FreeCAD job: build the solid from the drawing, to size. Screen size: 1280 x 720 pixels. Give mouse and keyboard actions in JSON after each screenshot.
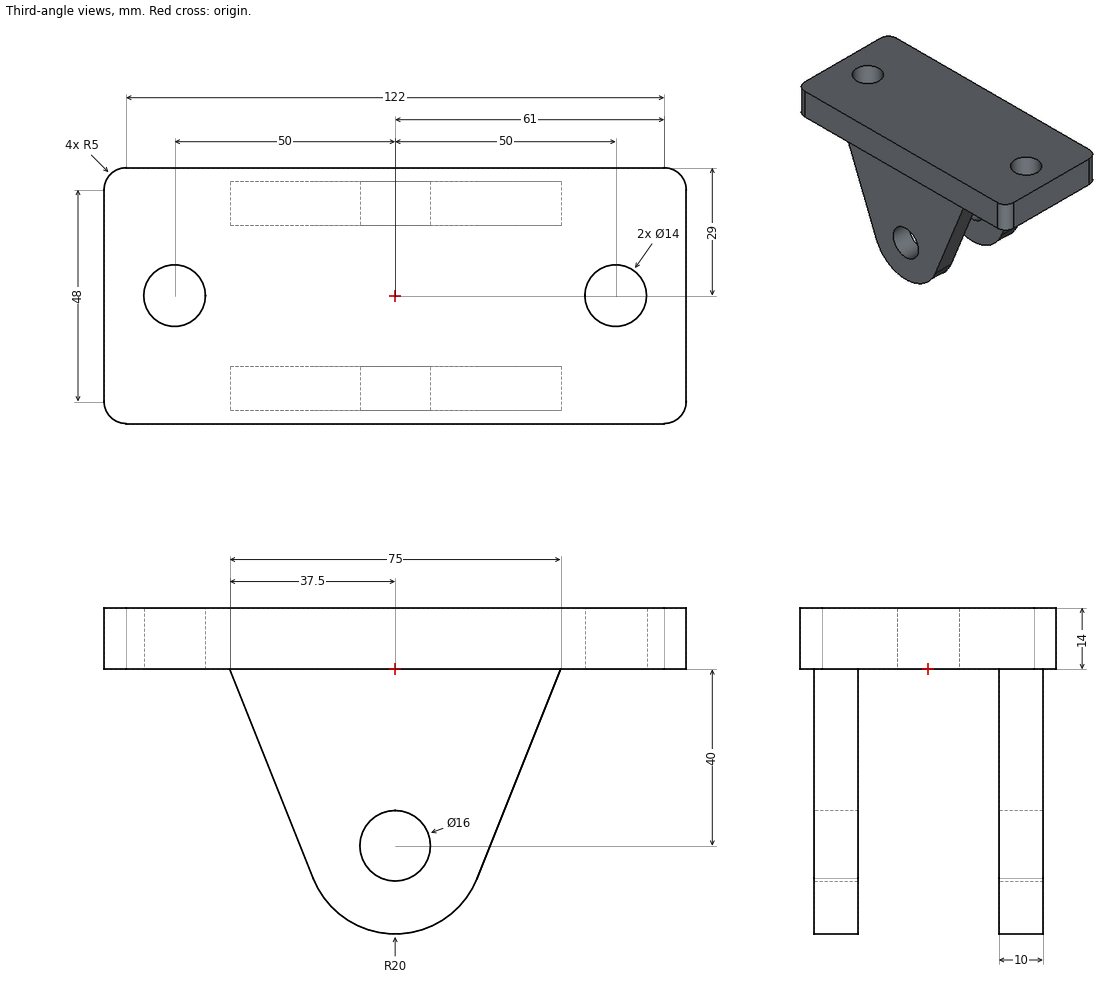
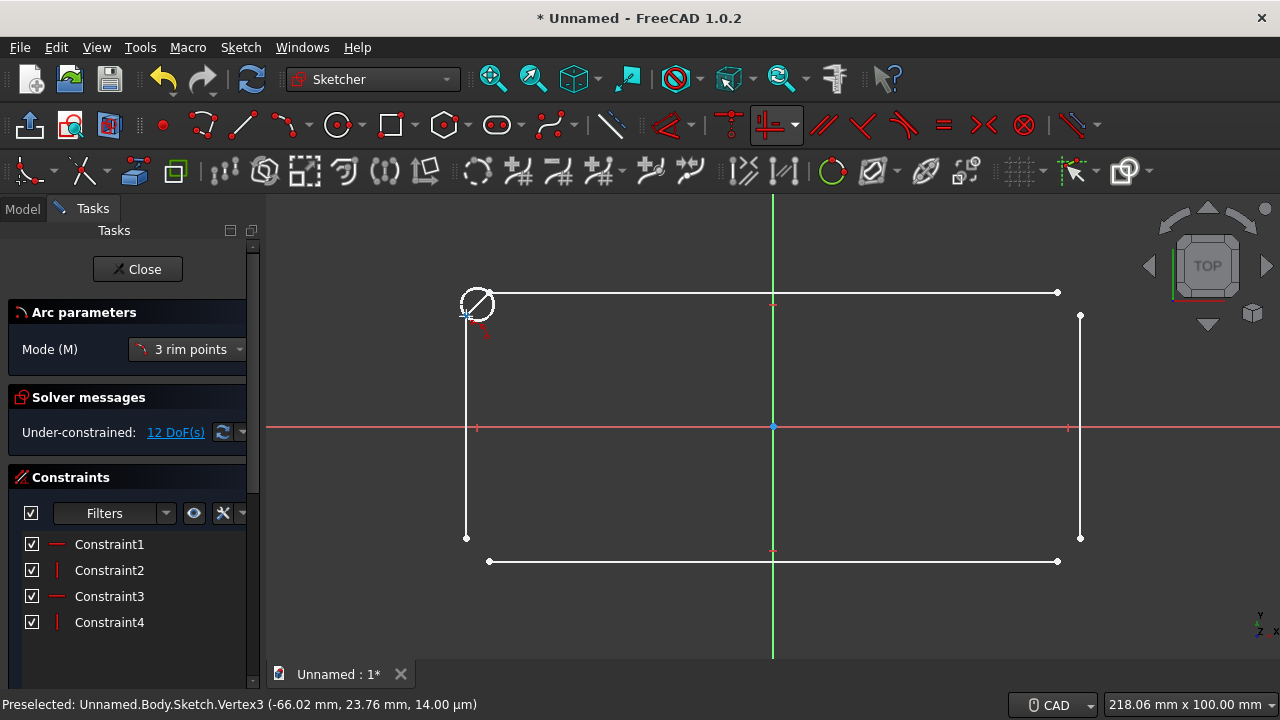
{"action": "scroll", "coordinate": [473, 298], "scroll_direction": "up", "scroll_amount": 5}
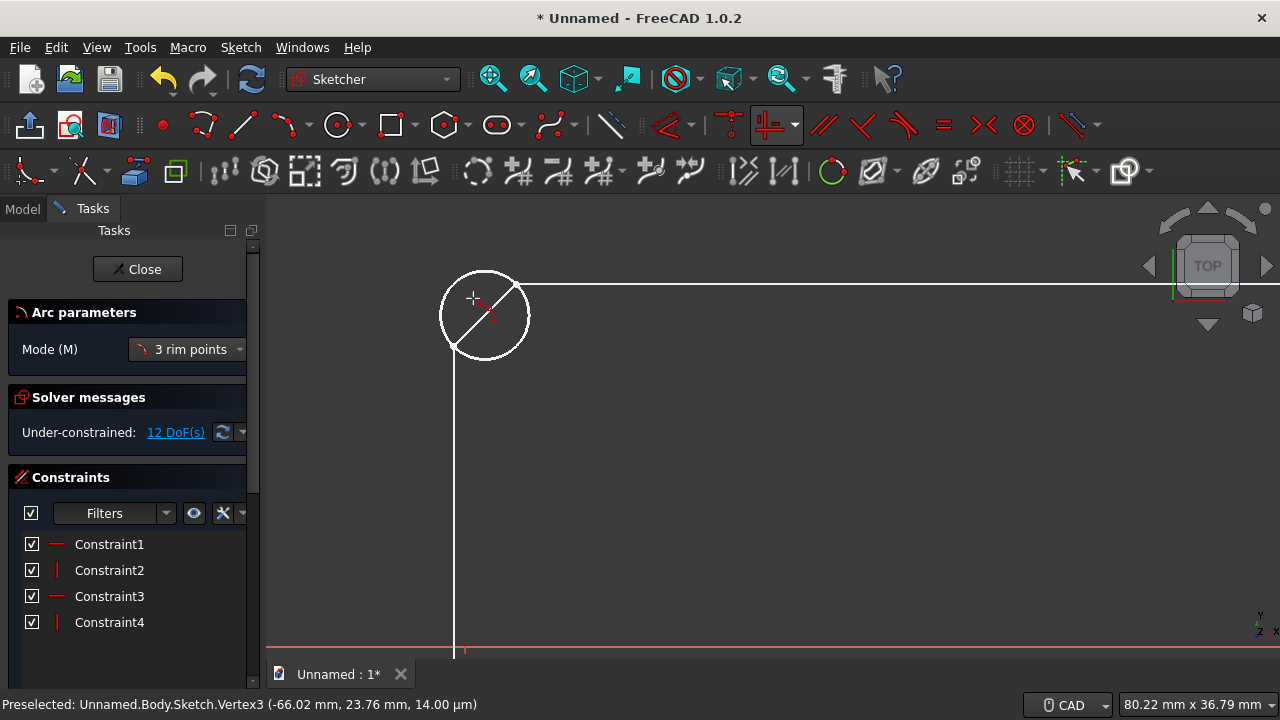
{"action": "left_click", "coordinate": [472, 299]}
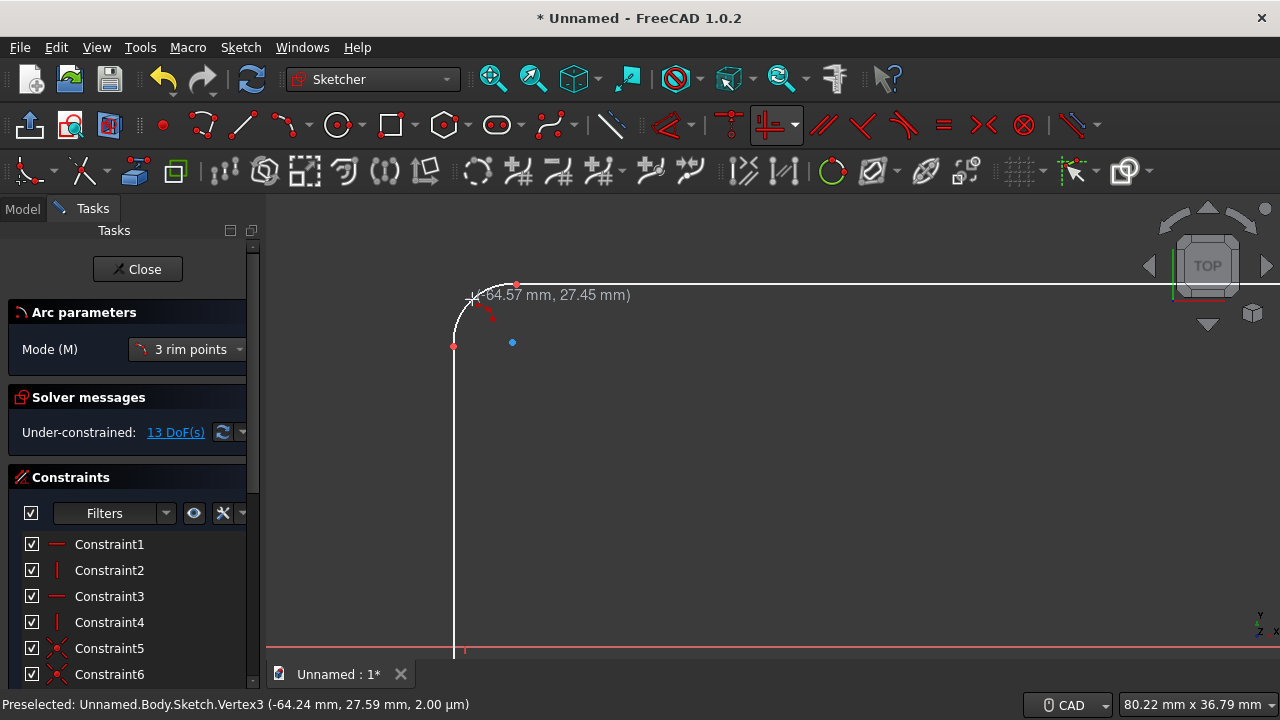
{"action": "scroll", "coordinate": [365, 298], "scroll_direction": "down", "scroll_amount": 5}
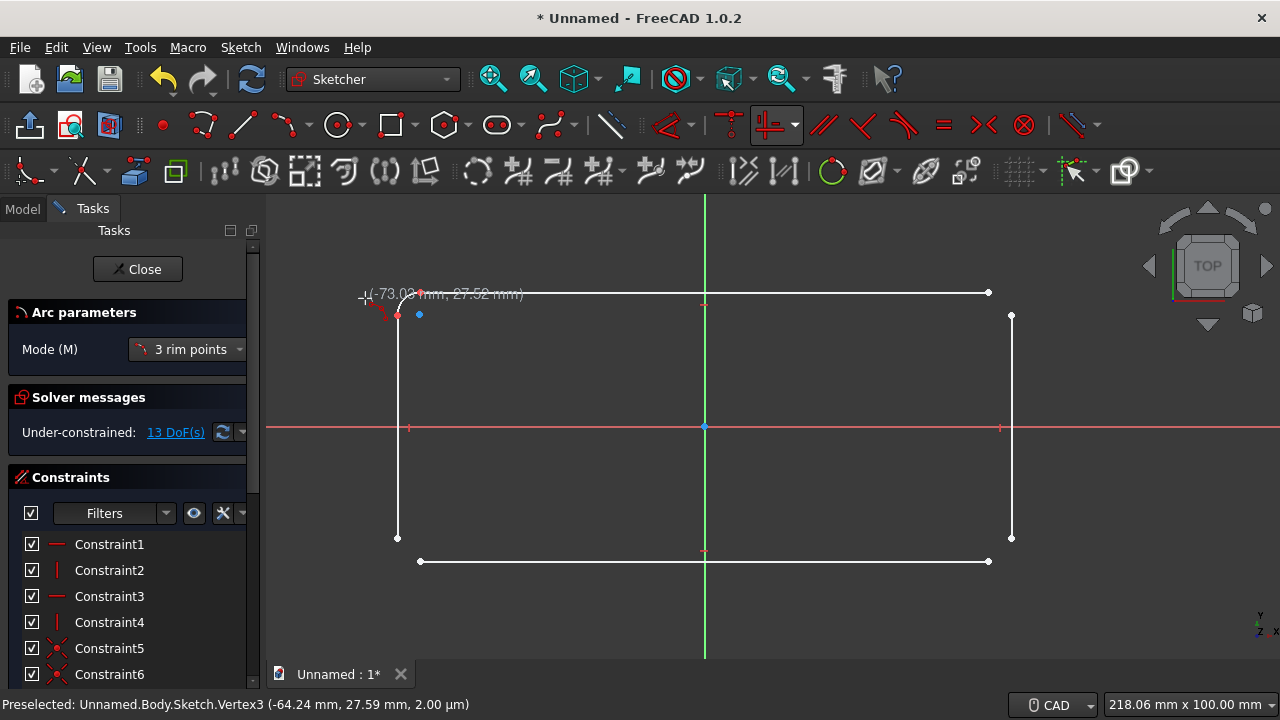
{"action": "left_click", "coordinate": [398, 539]}
{"action": "left_click", "coordinate": [421, 562]}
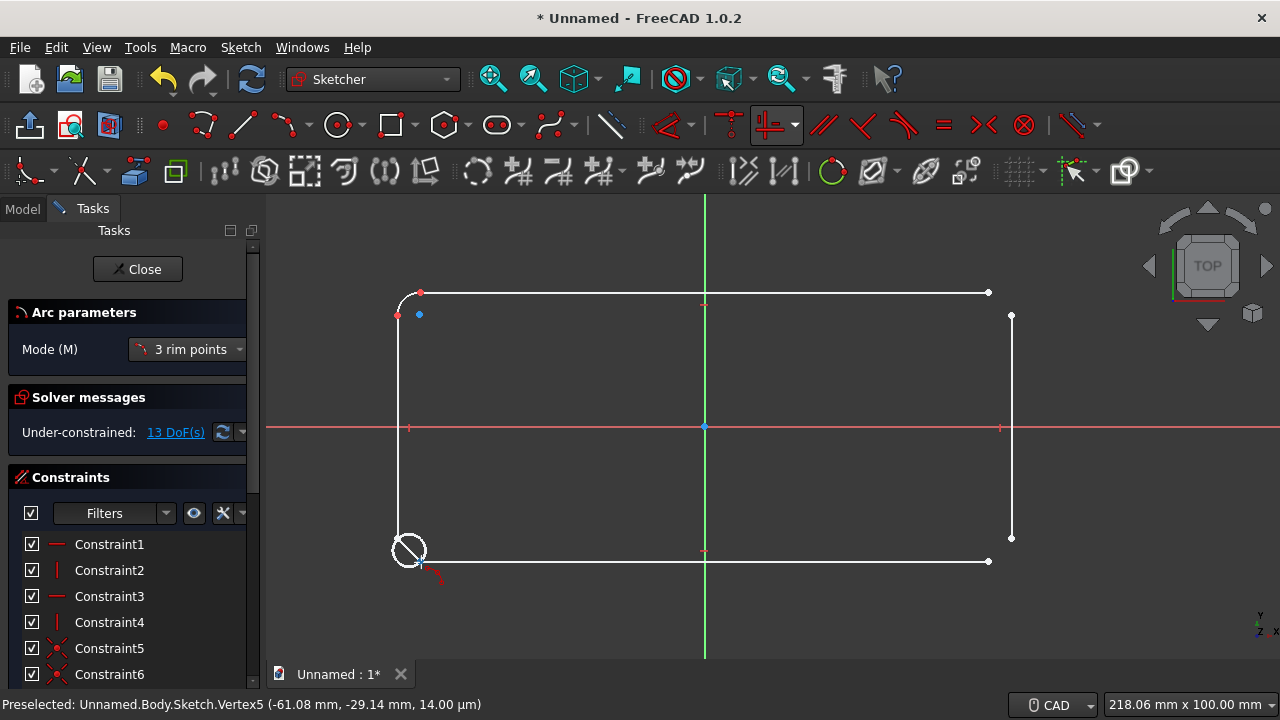
{"action": "scroll", "coordinate": [405, 555], "scroll_direction": "up", "scroll_amount": 5}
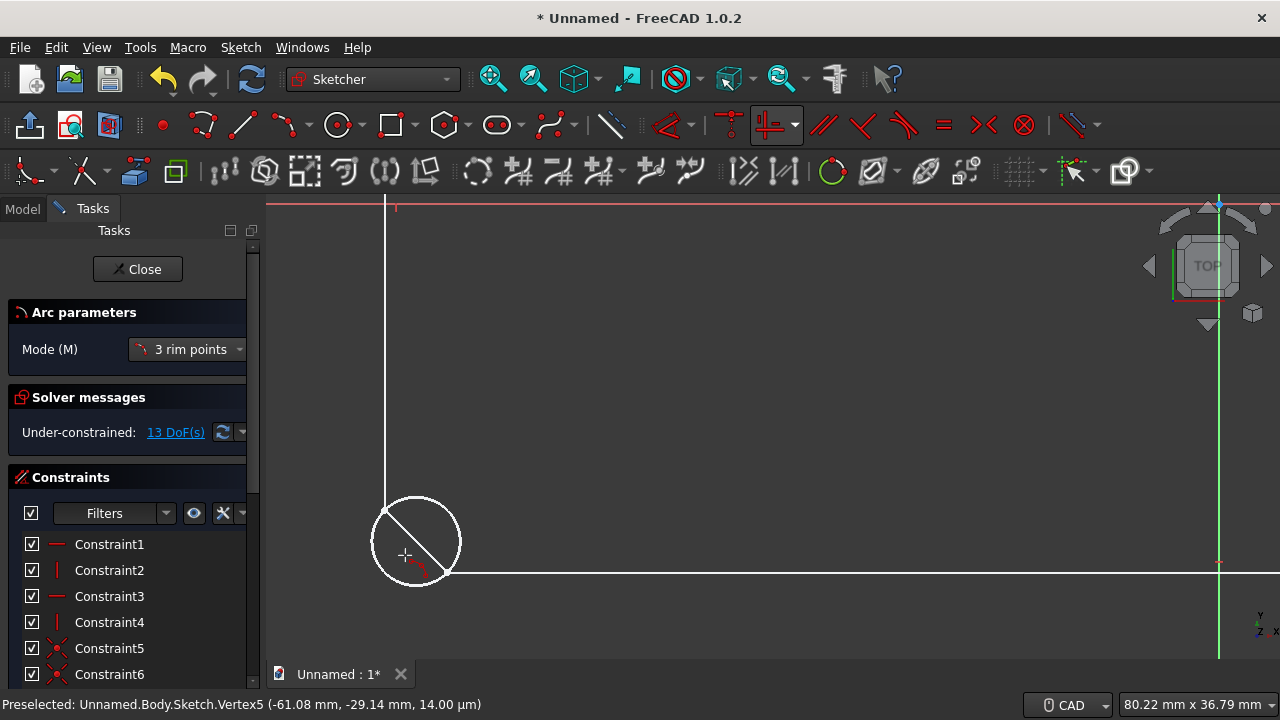
{"action": "left_click", "coordinate": [404, 552]}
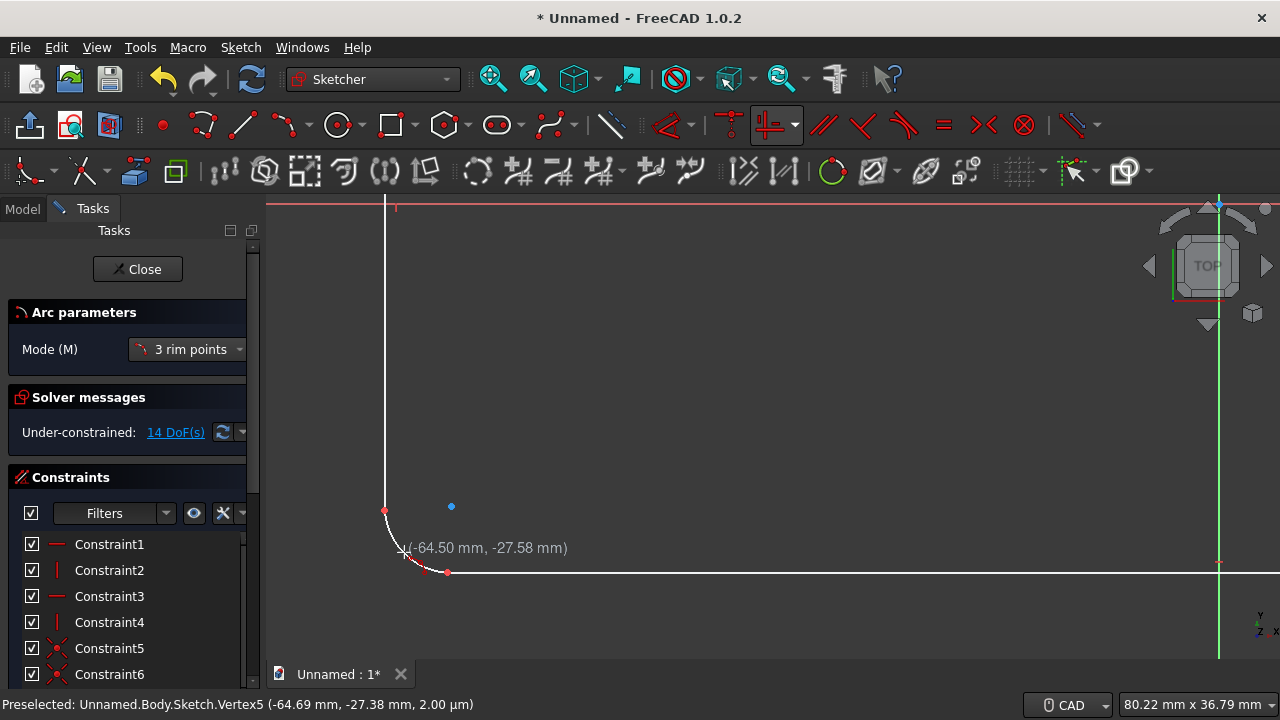
{"action": "scroll", "coordinate": [405, 556], "scroll_direction": "down", "scroll_amount": 5}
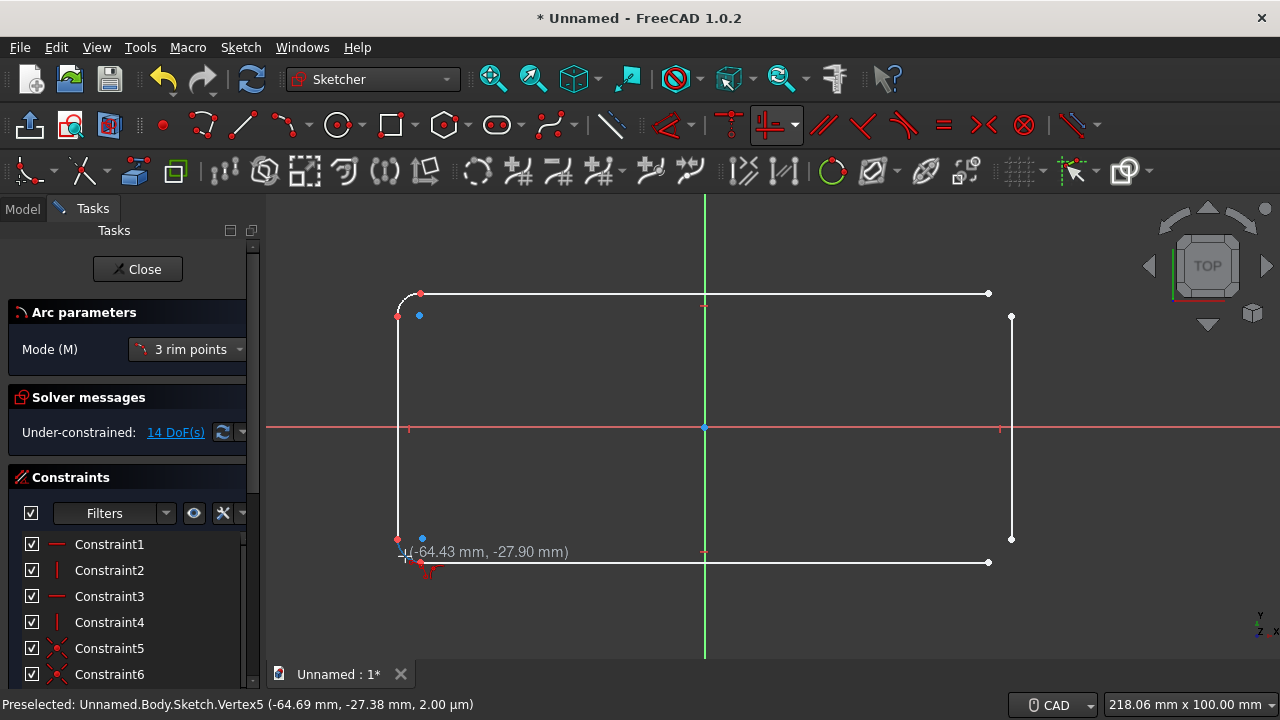
{"action": "left_click", "coordinate": [989, 563]}
{"action": "left_click", "coordinate": [1012, 540]}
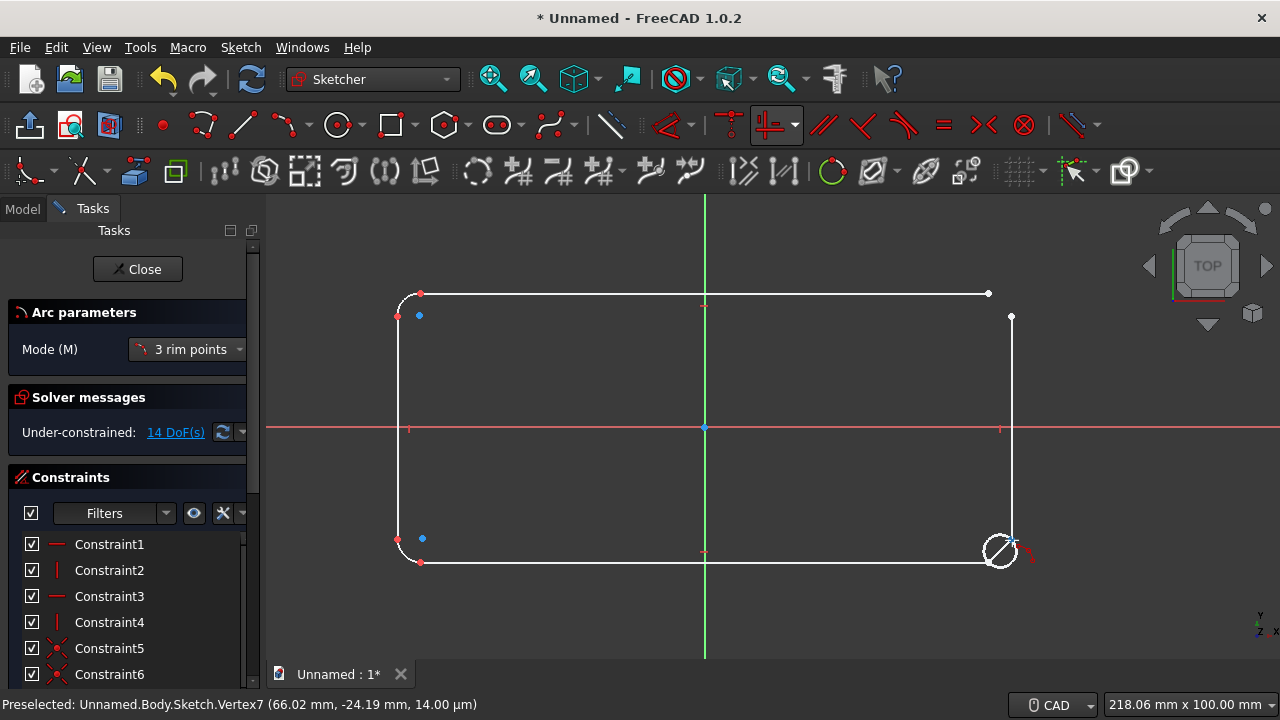
{"action": "scroll", "coordinate": [1005, 555], "scroll_direction": "up", "scroll_amount": 5}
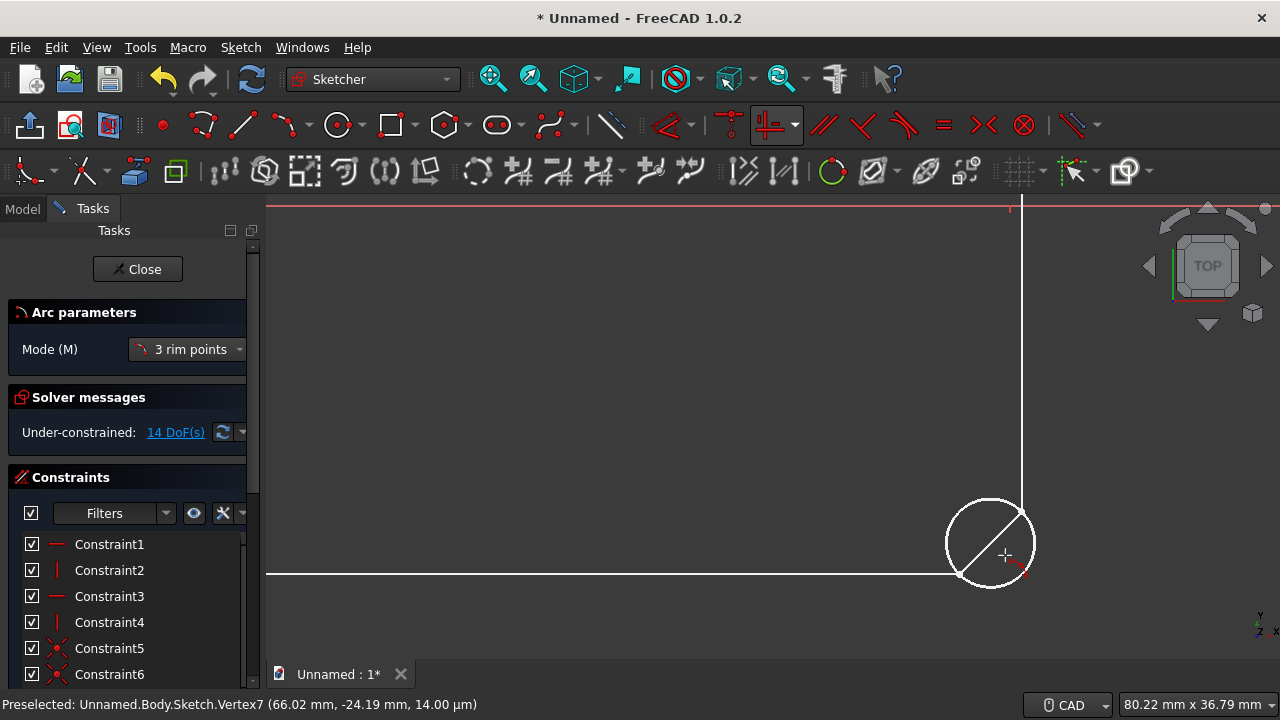
{"action": "left_click", "coordinate": [1003, 554]}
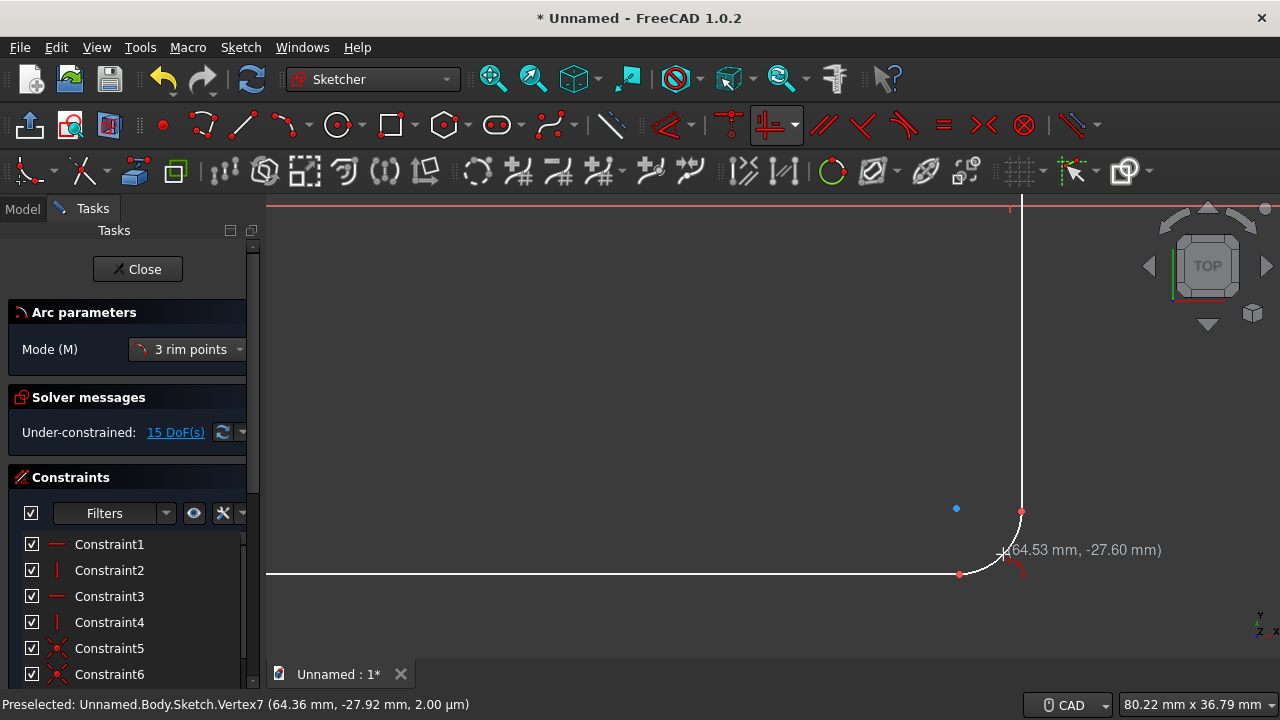
{"action": "scroll", "coordinate": [1005, 555], "scroll_direction": "down", "scroll_amount": 5}